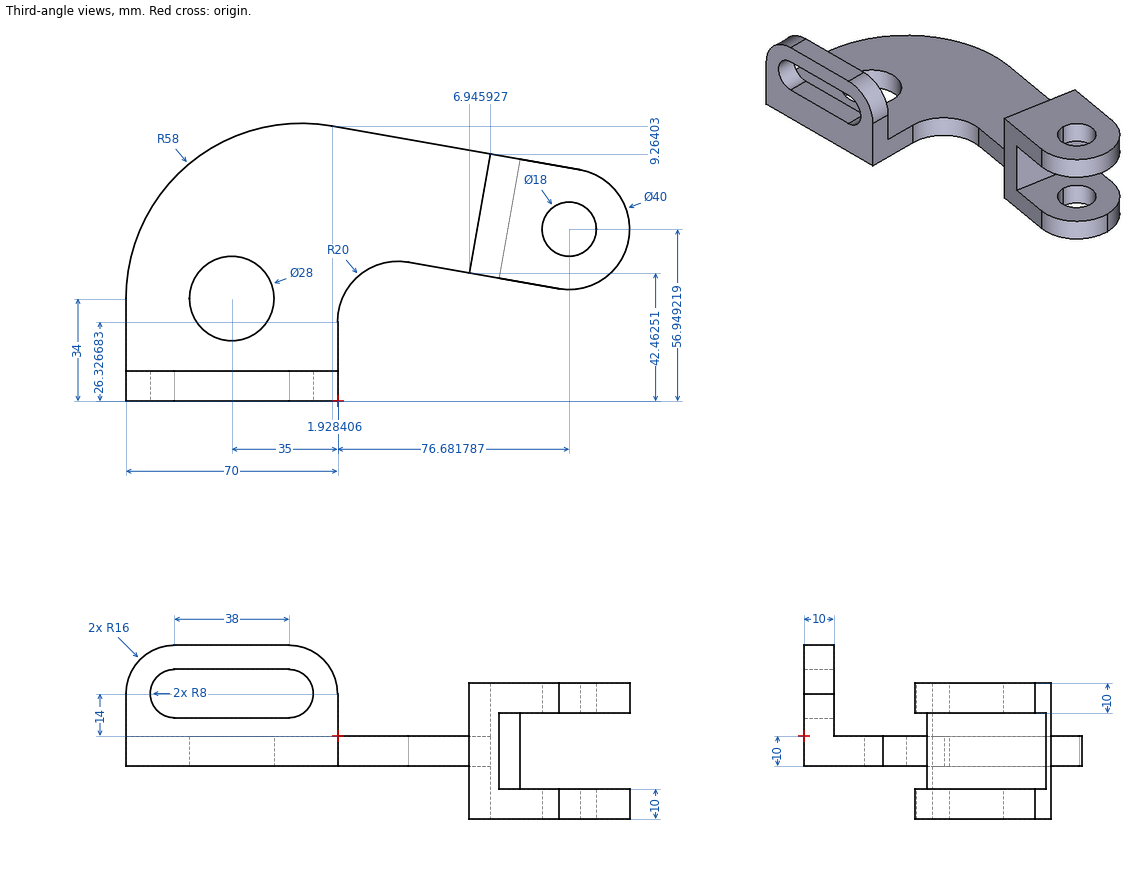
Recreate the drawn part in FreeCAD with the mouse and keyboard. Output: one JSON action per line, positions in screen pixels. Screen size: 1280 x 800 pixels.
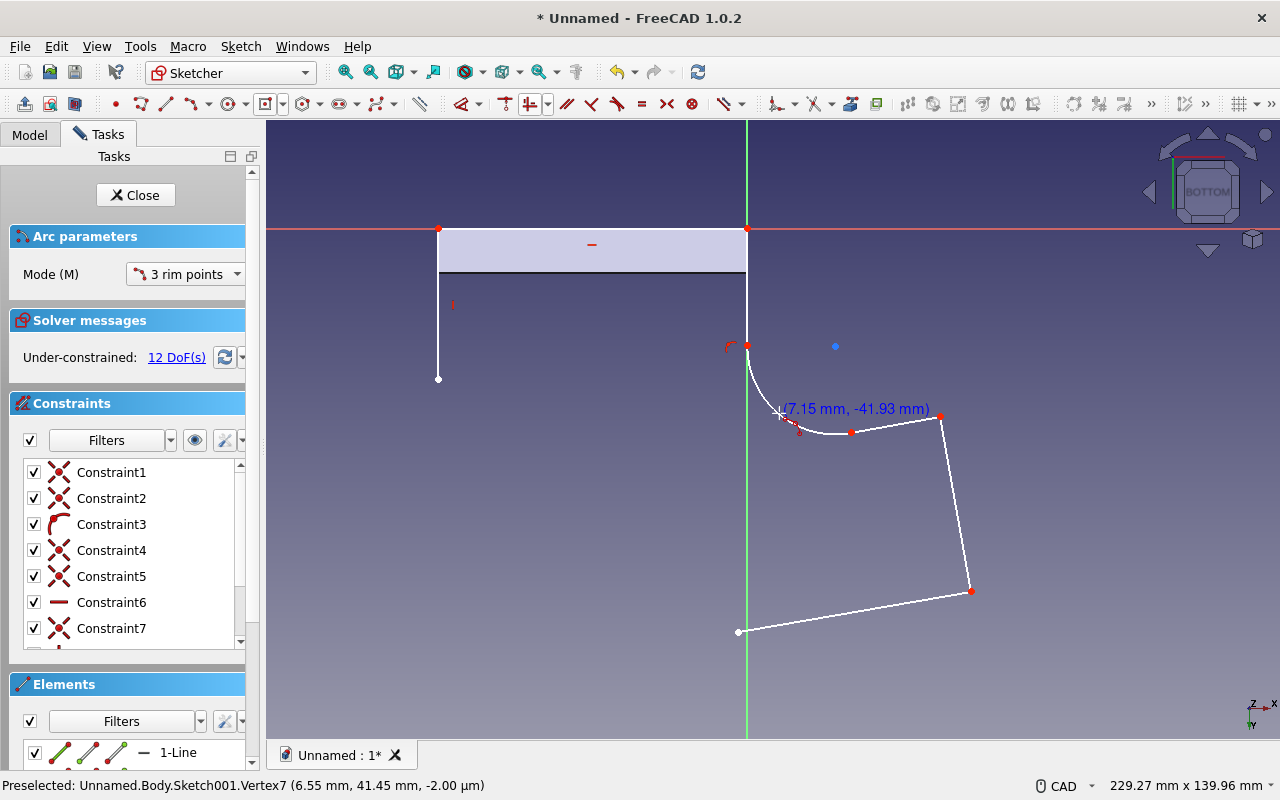
{"action": "left_click", "coordinate": [438, 380]}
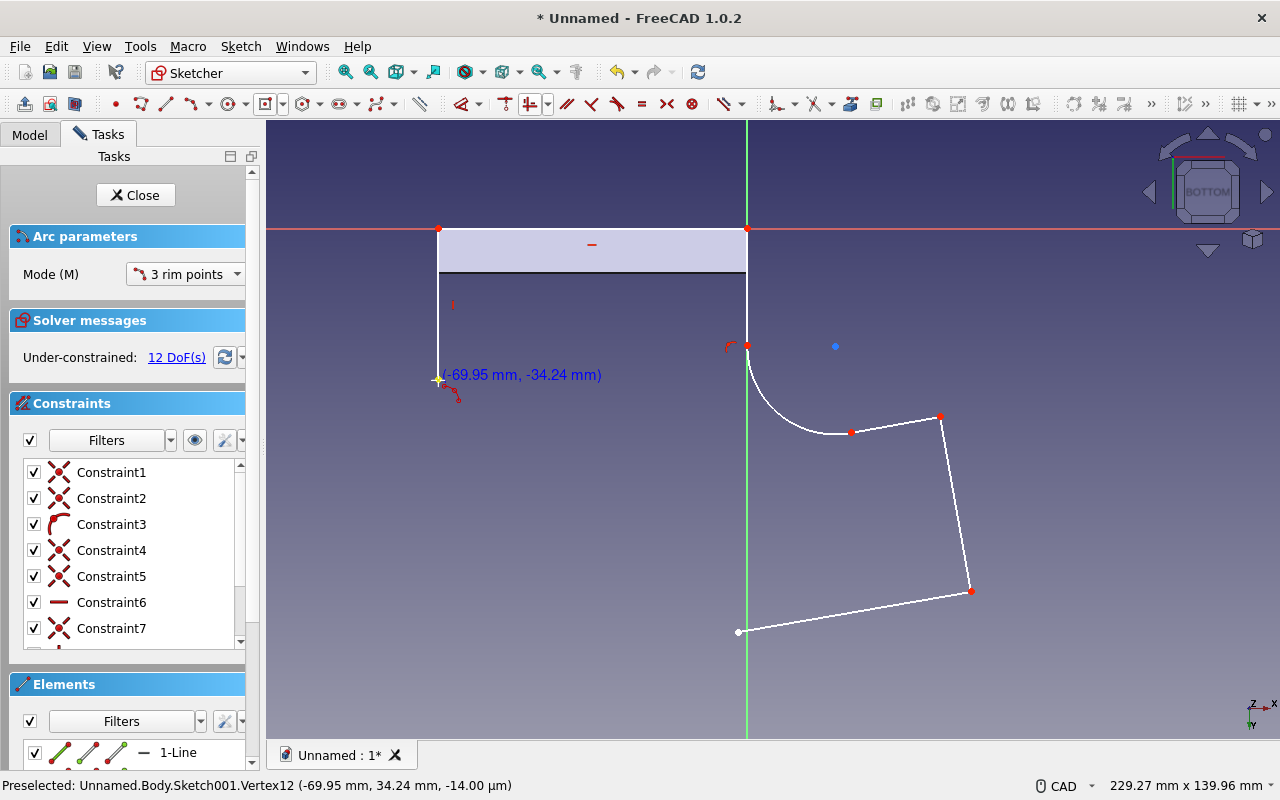
{"action": "scroll", "coordinate": [739, 632], "scroll_direction": "up", "scroll_amount": 4}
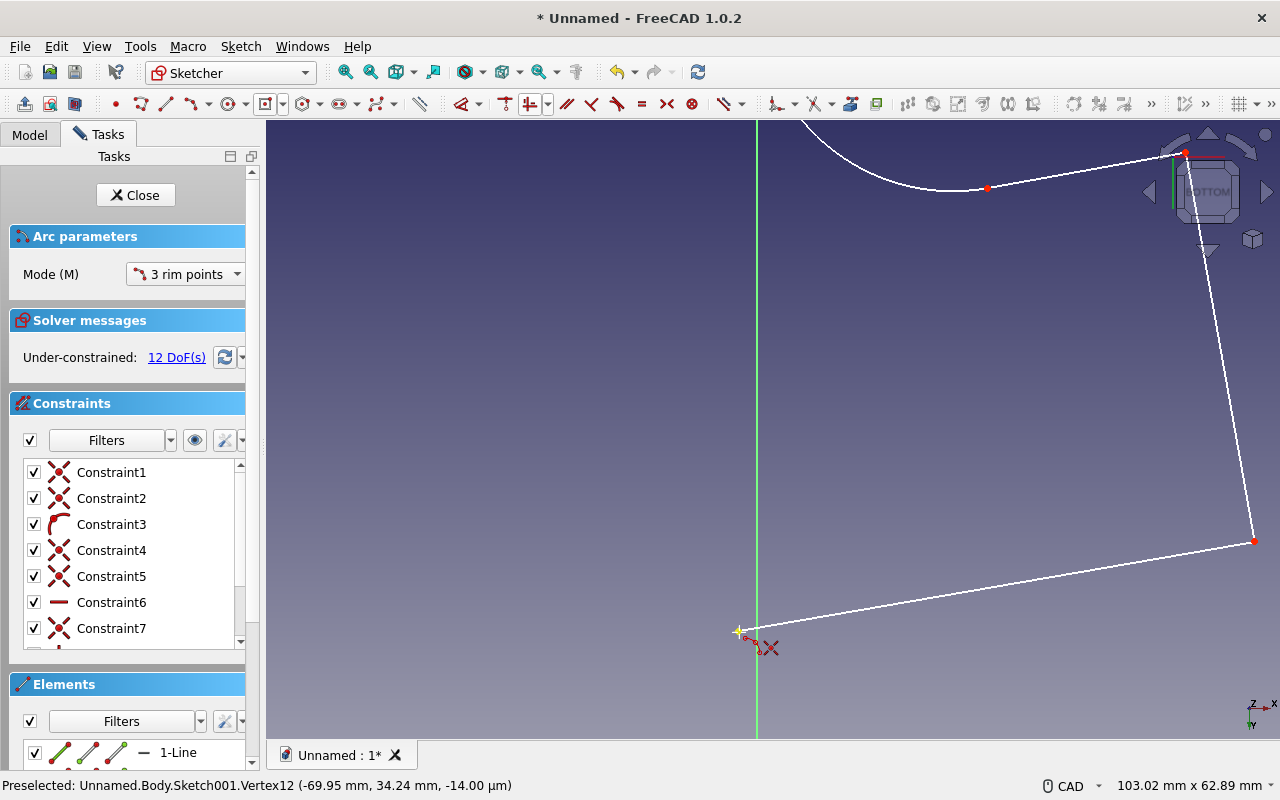
{"action": "left_click", "coordinate": [738, 631]}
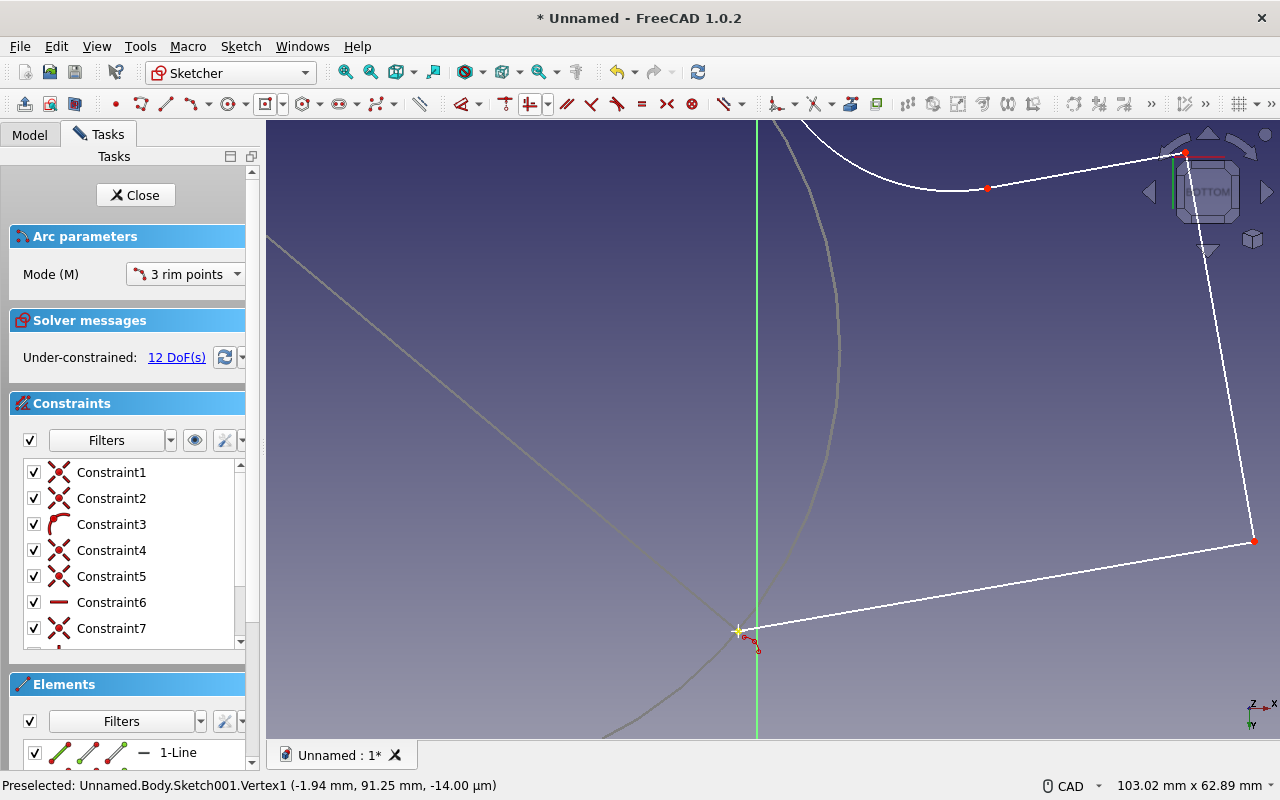
{"action": "scroll", "coordinate": [739, 632], "scroll_direction": "down", "scroll_amount": 4}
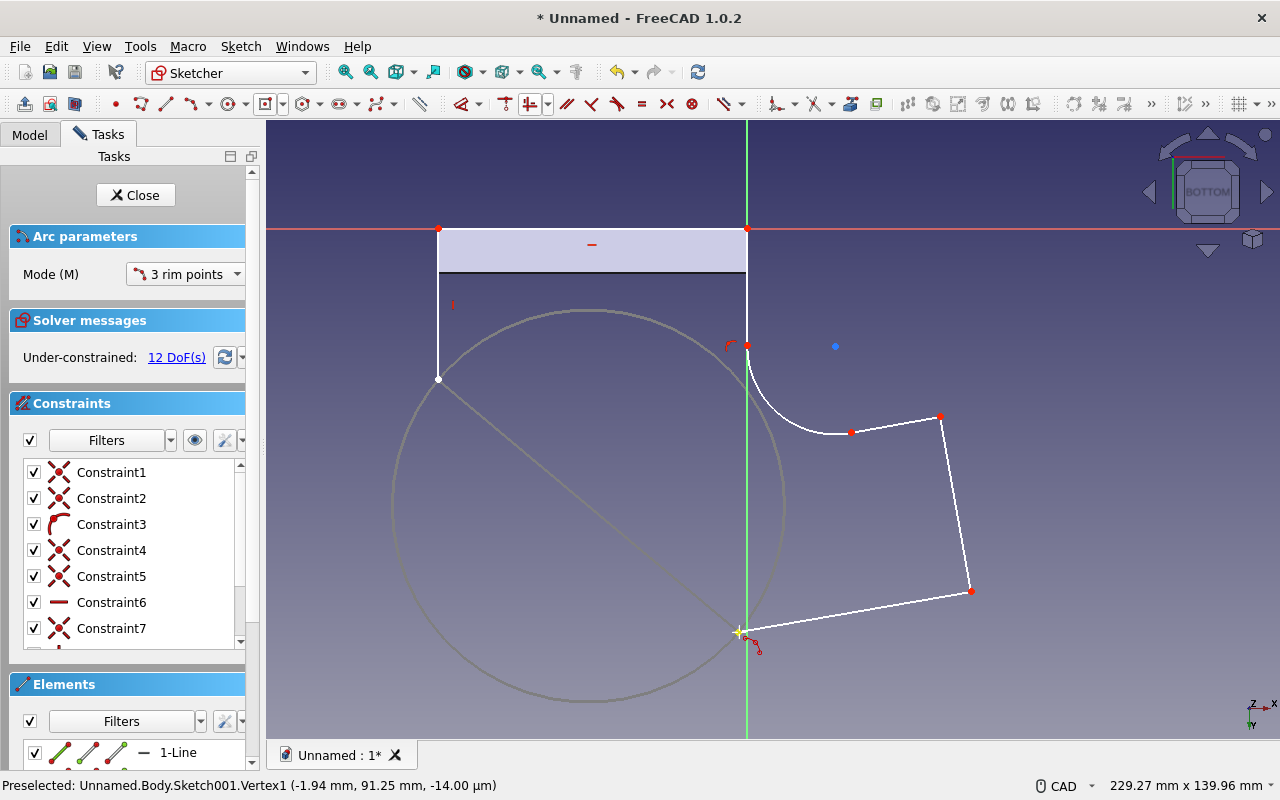
{"action": "left_click", "coordinate": [529, 575]}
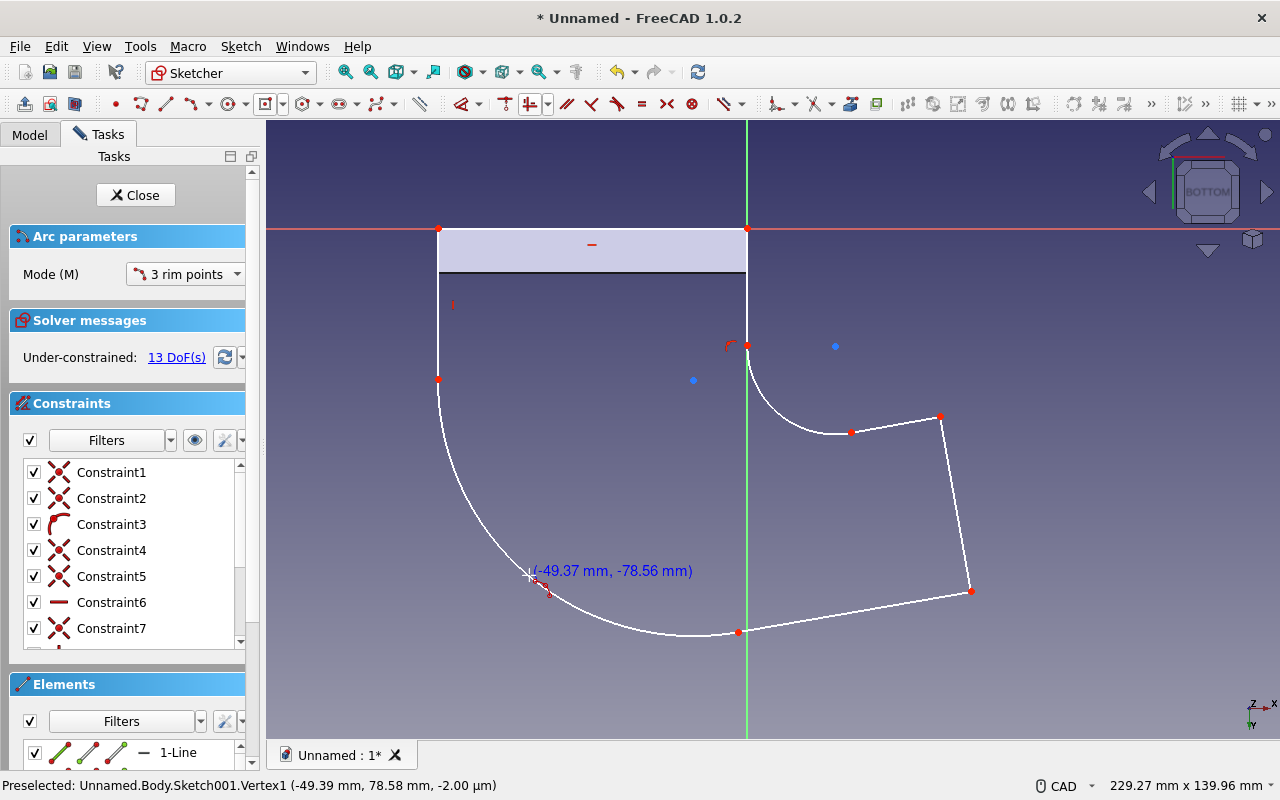
{"action": "key", "text": "g c"}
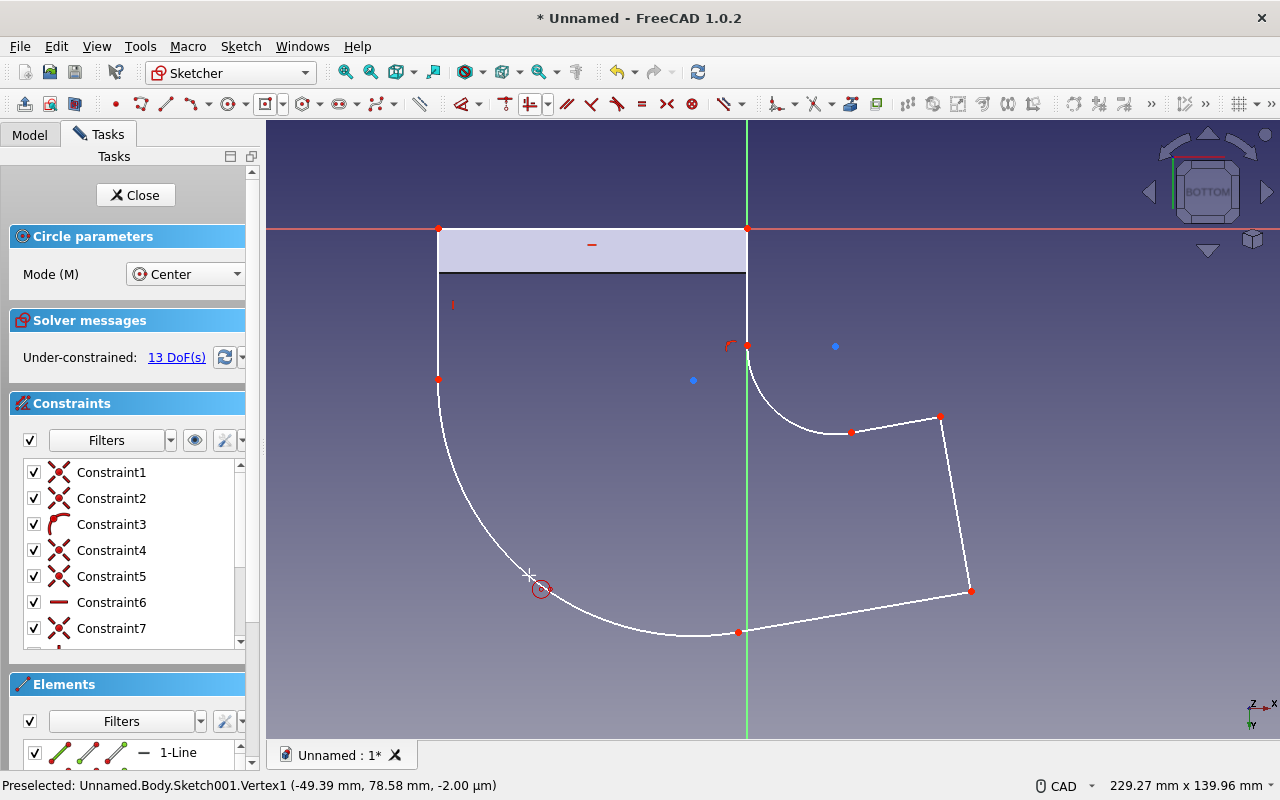
{"action": "left_click", "coordinate": [593, 379]}
{"action": "left_click", "coordinate": [636, 335]}
{"action": "key", "text": "Escape"}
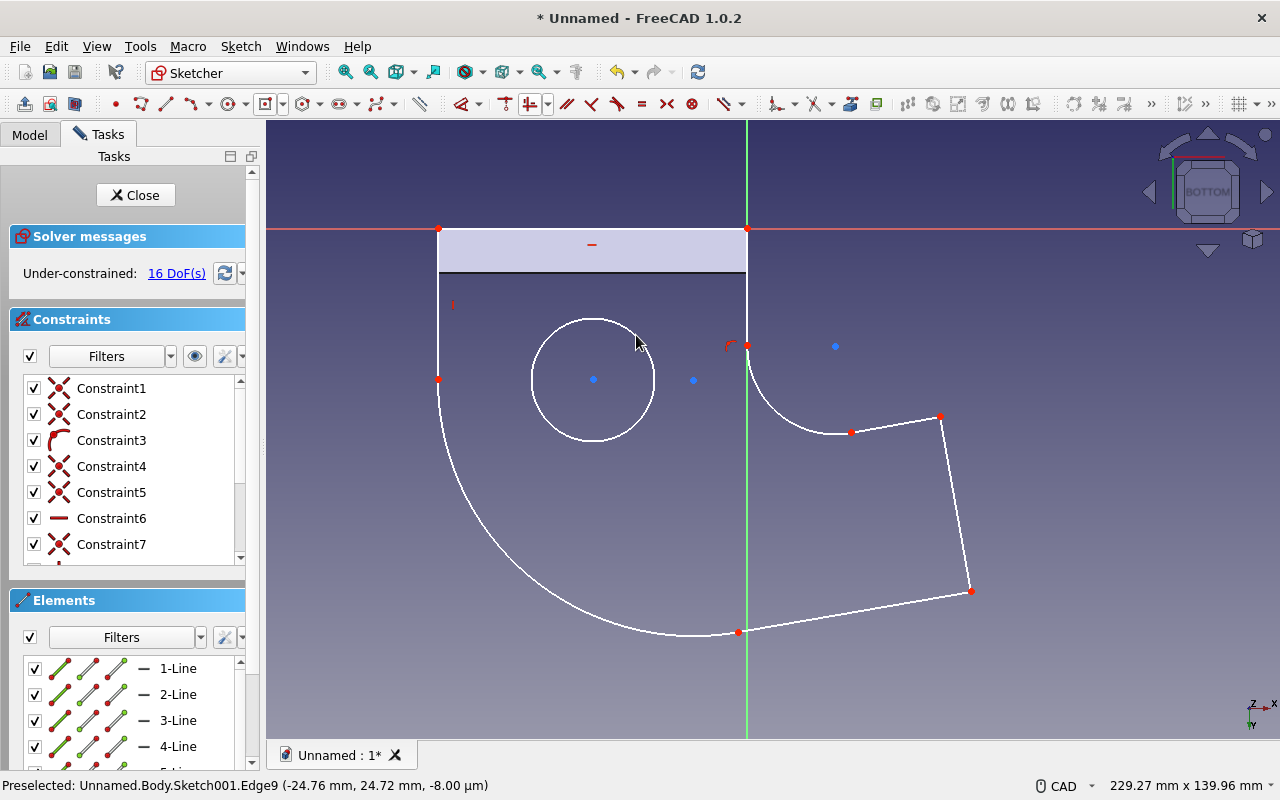
{"action": "left_click", "coordinate": [808, 620]}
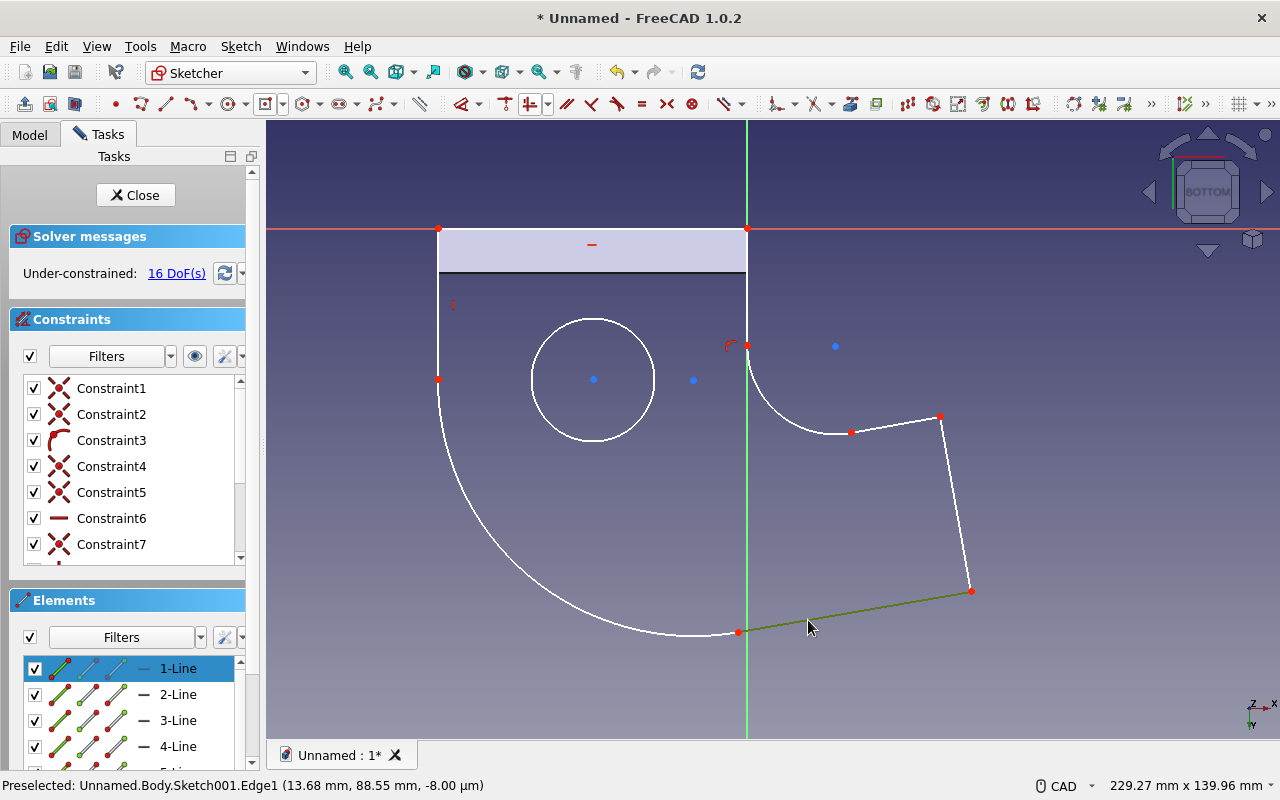
{"action": "left_click", "coordinate": [472, 508]}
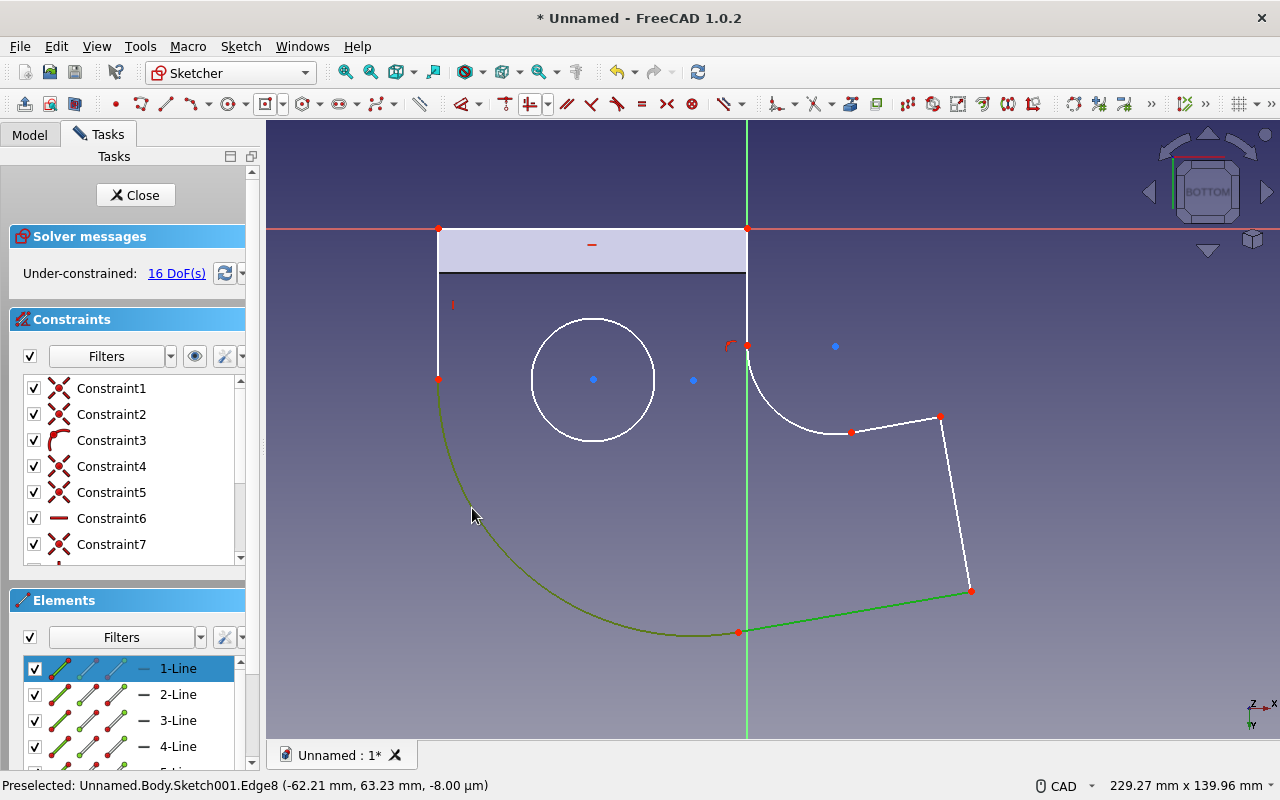
{"action": "left_click", "coordinate": [617, 104]}